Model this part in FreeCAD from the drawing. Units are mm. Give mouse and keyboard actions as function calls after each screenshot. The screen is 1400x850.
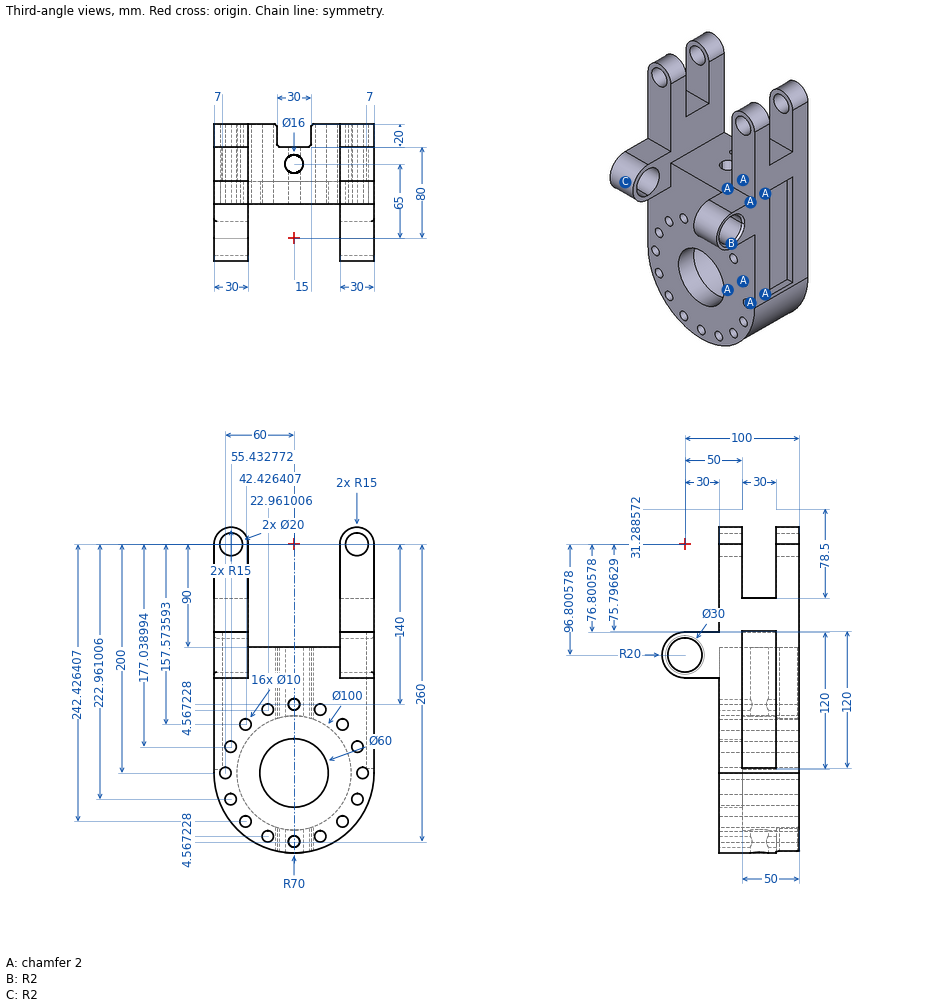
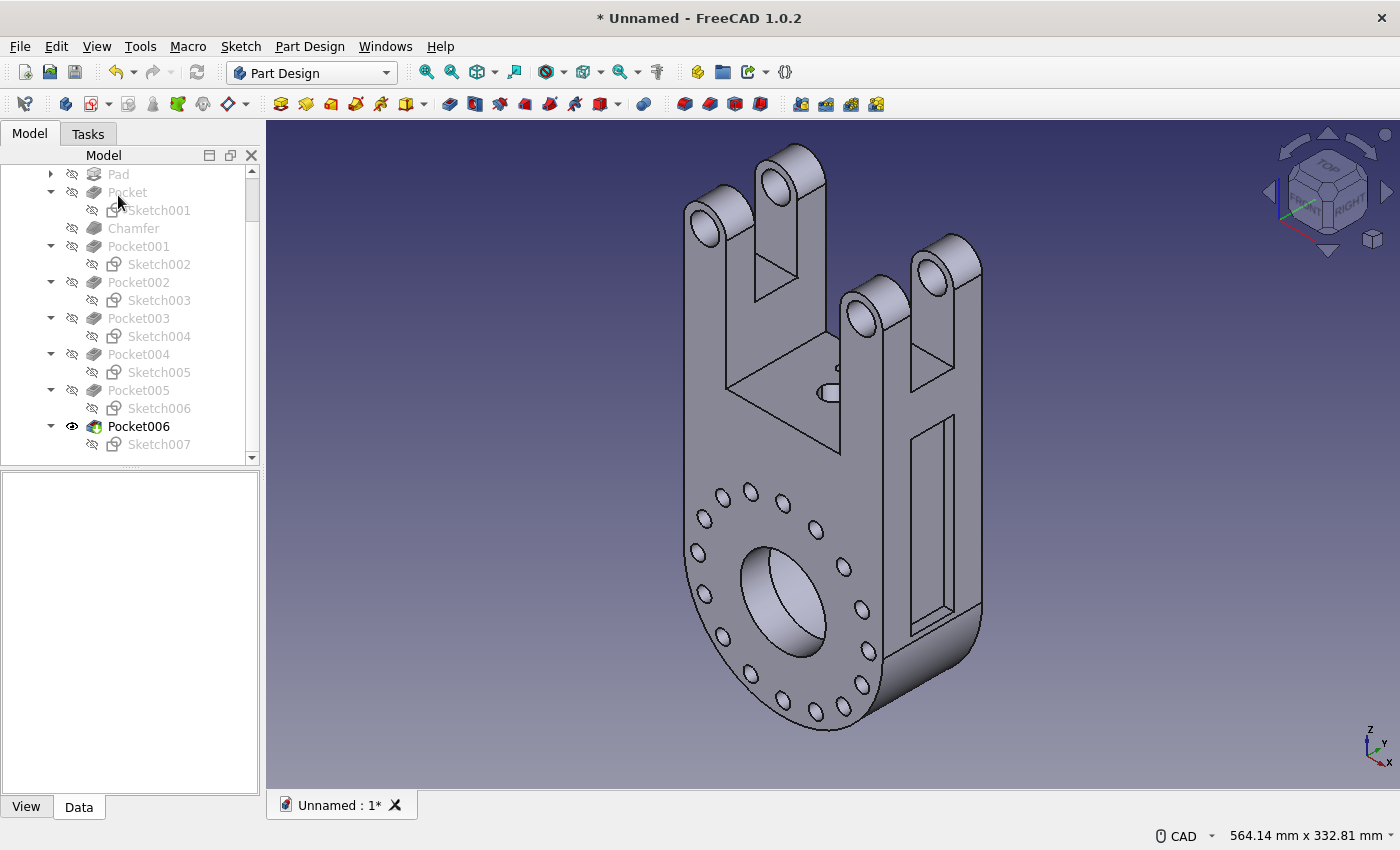
key(6)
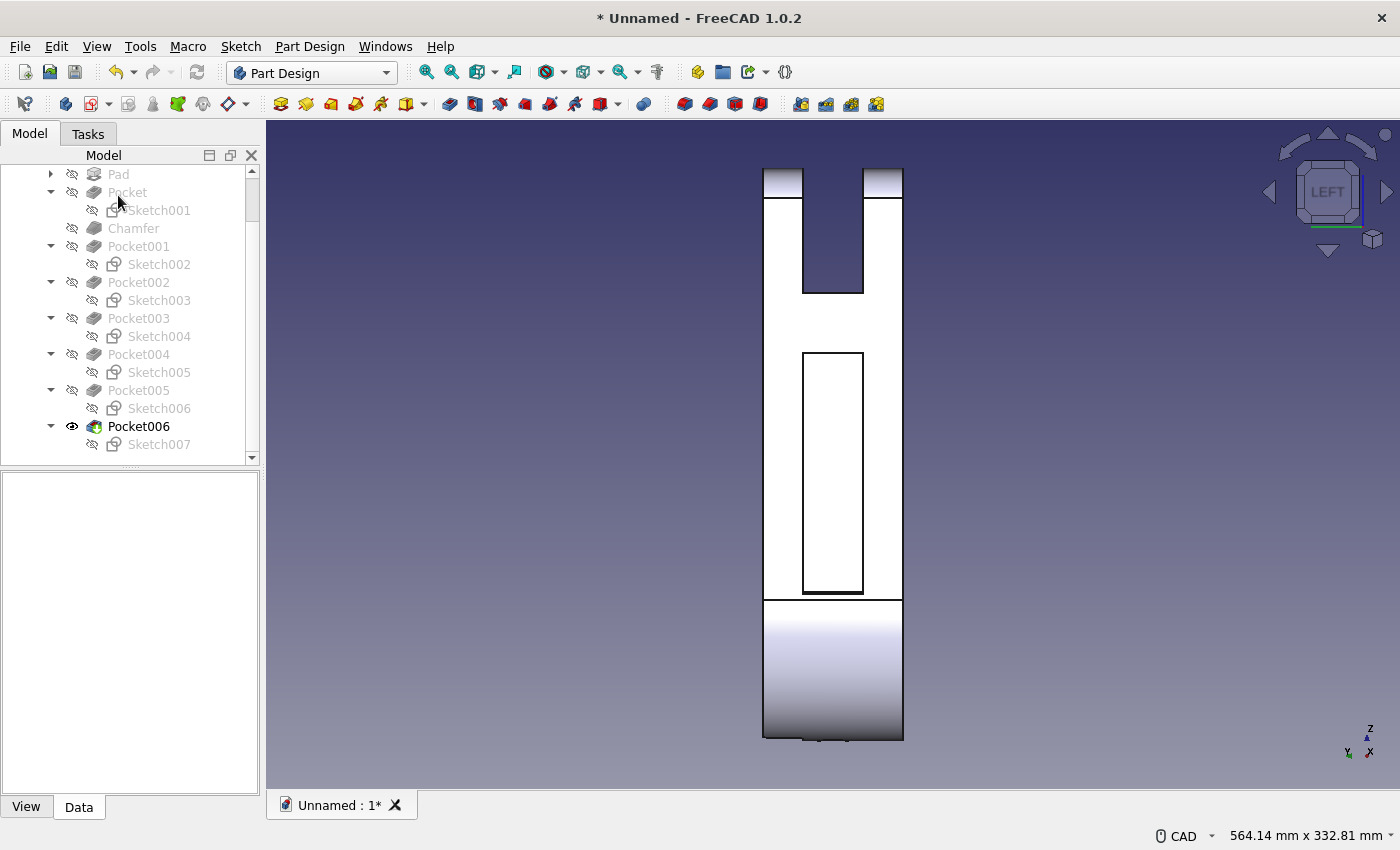
click(793, 341)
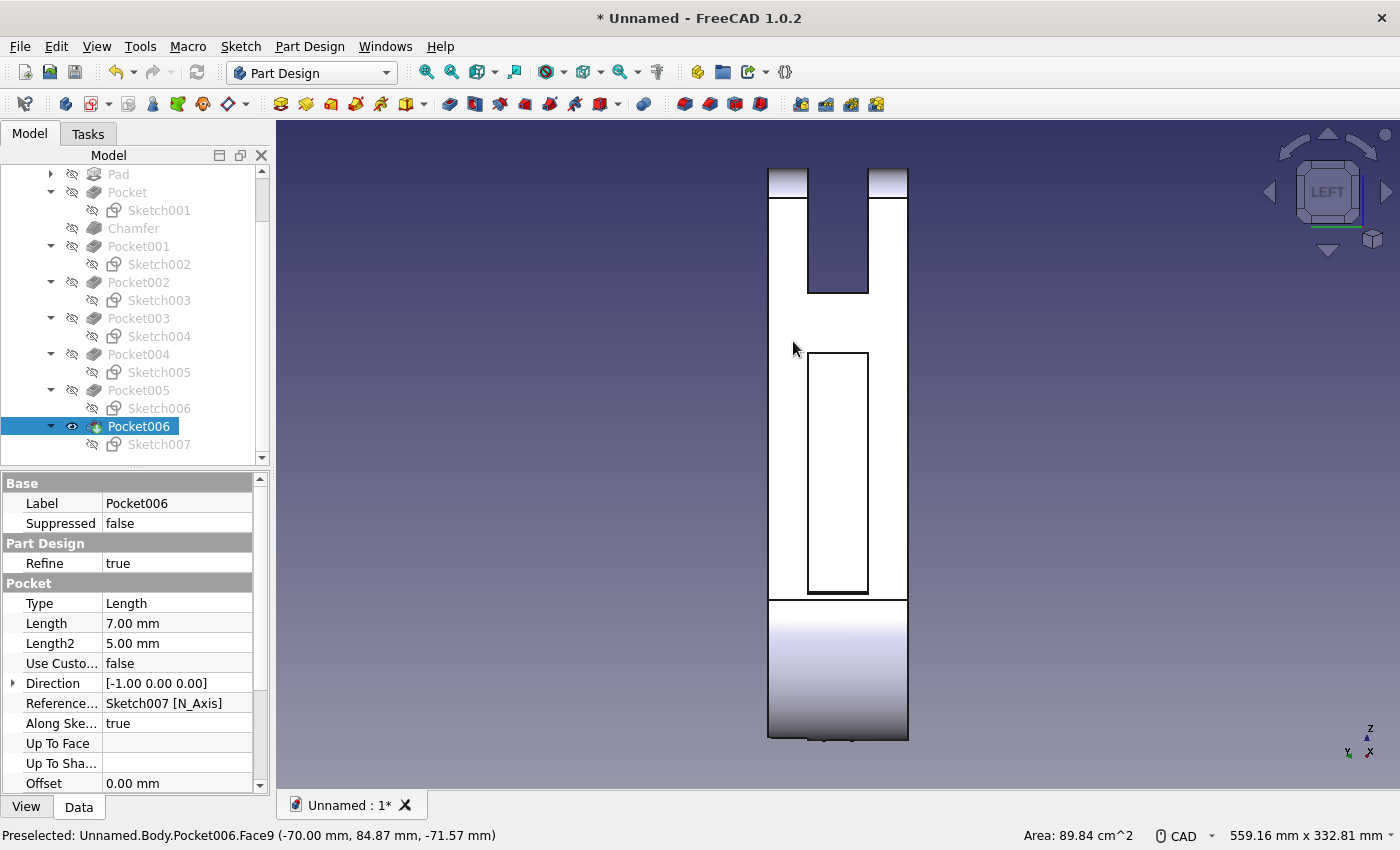
click(90, 104)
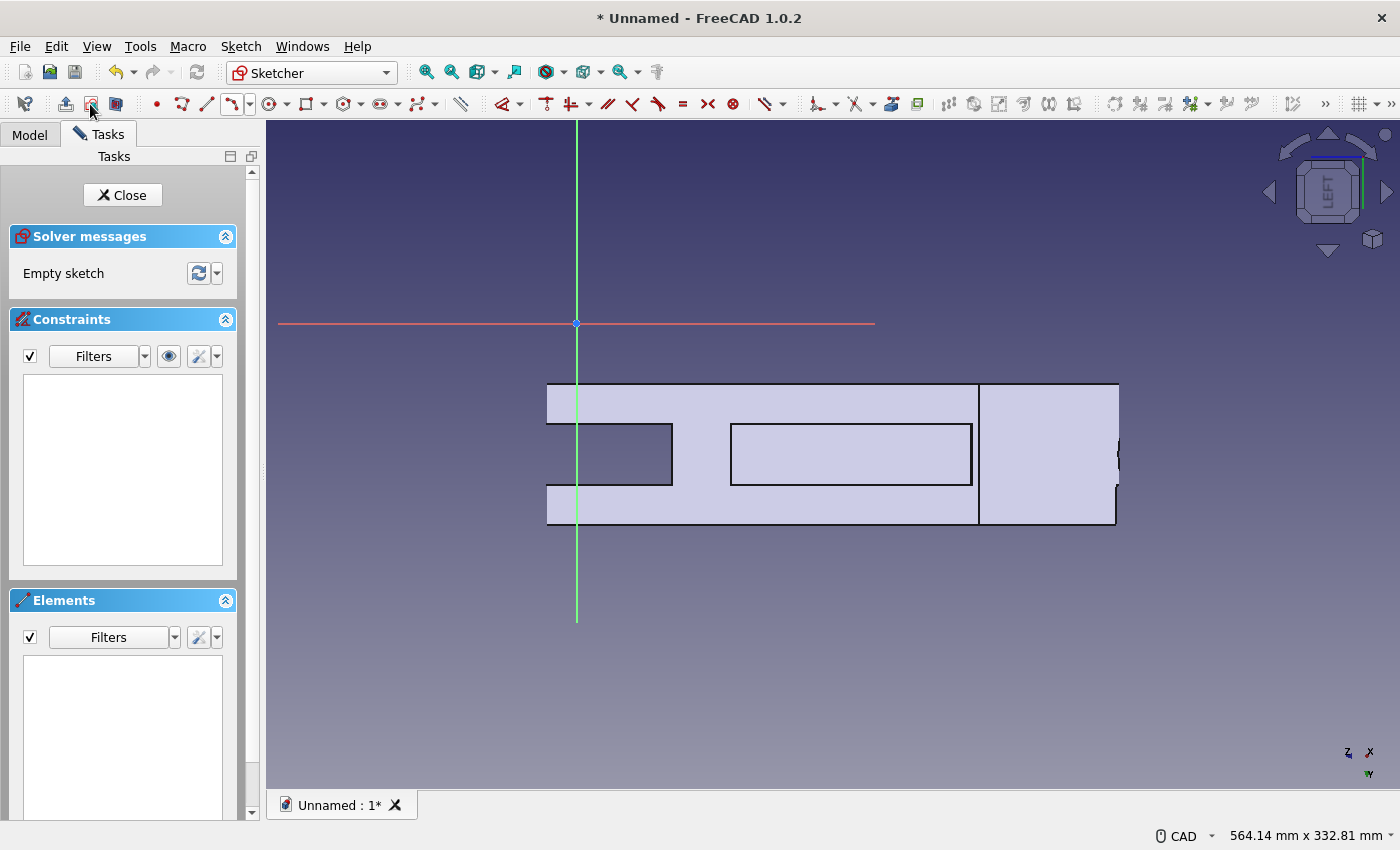
scroll(653, 296, up, 5)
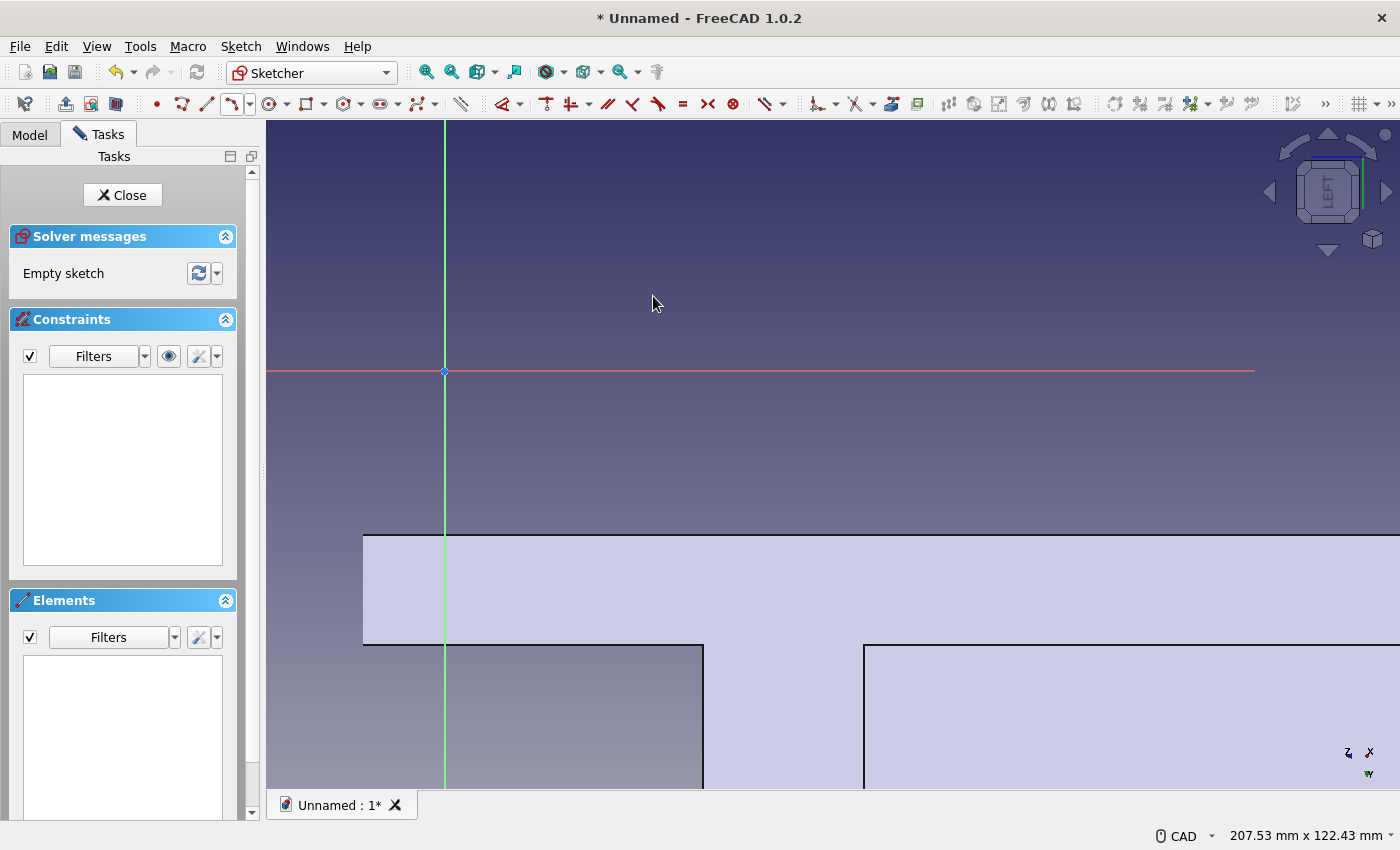
key(g)
key(m)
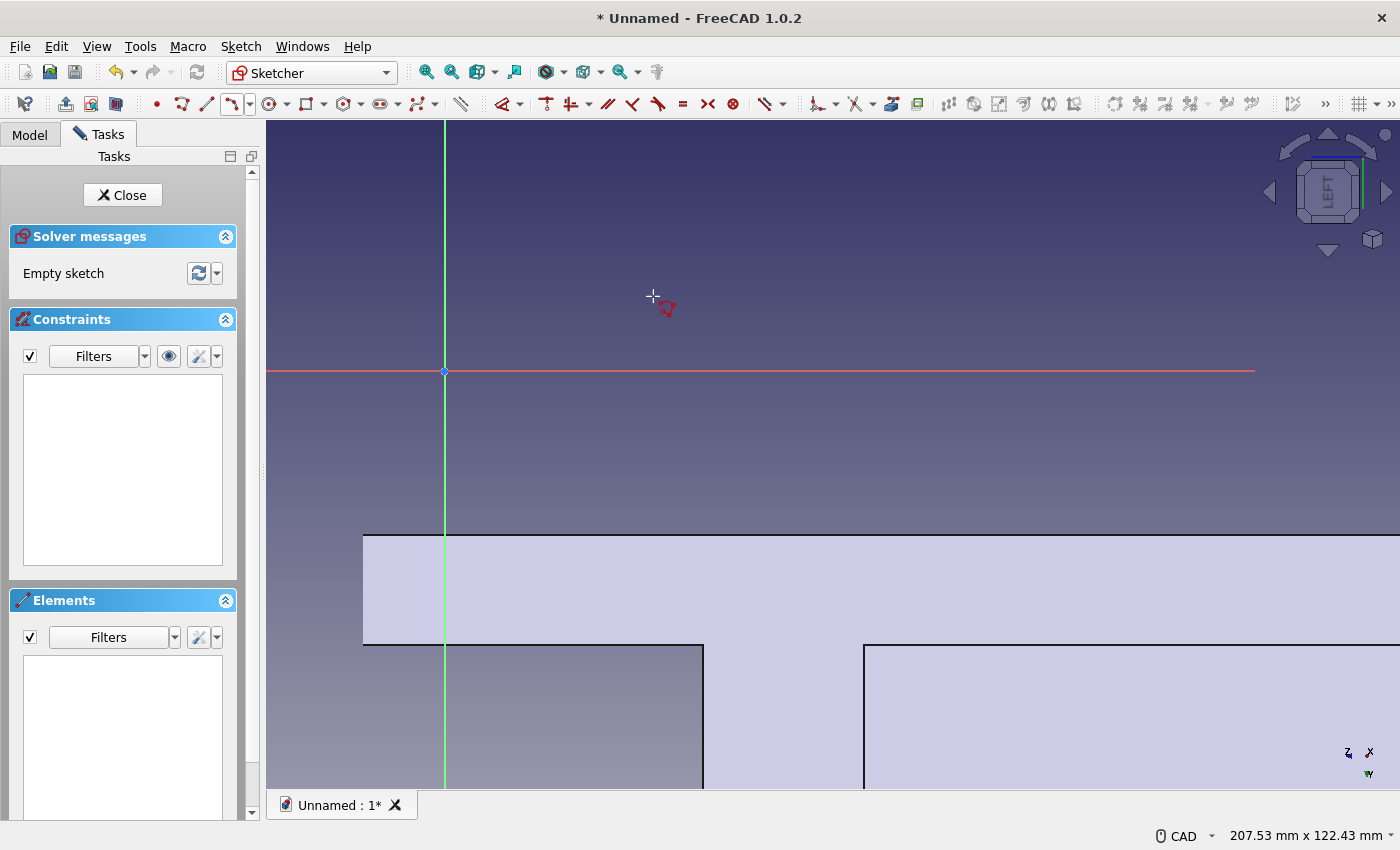
click(864, 371)
click(864, 645)
click(1083, 645)
click(1083, 371)
right_click(1083, 371)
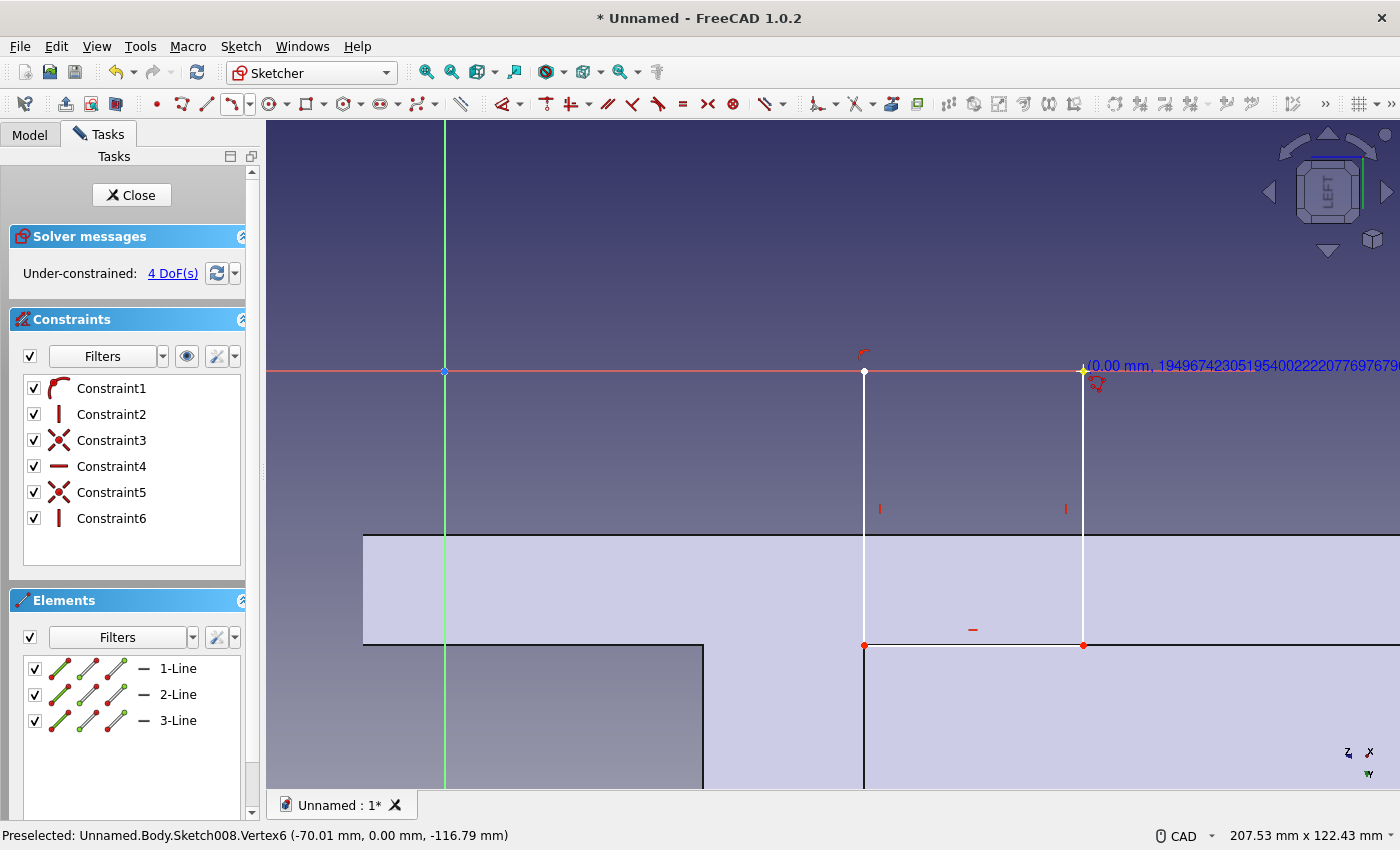
key(g)
key(3)
key(a)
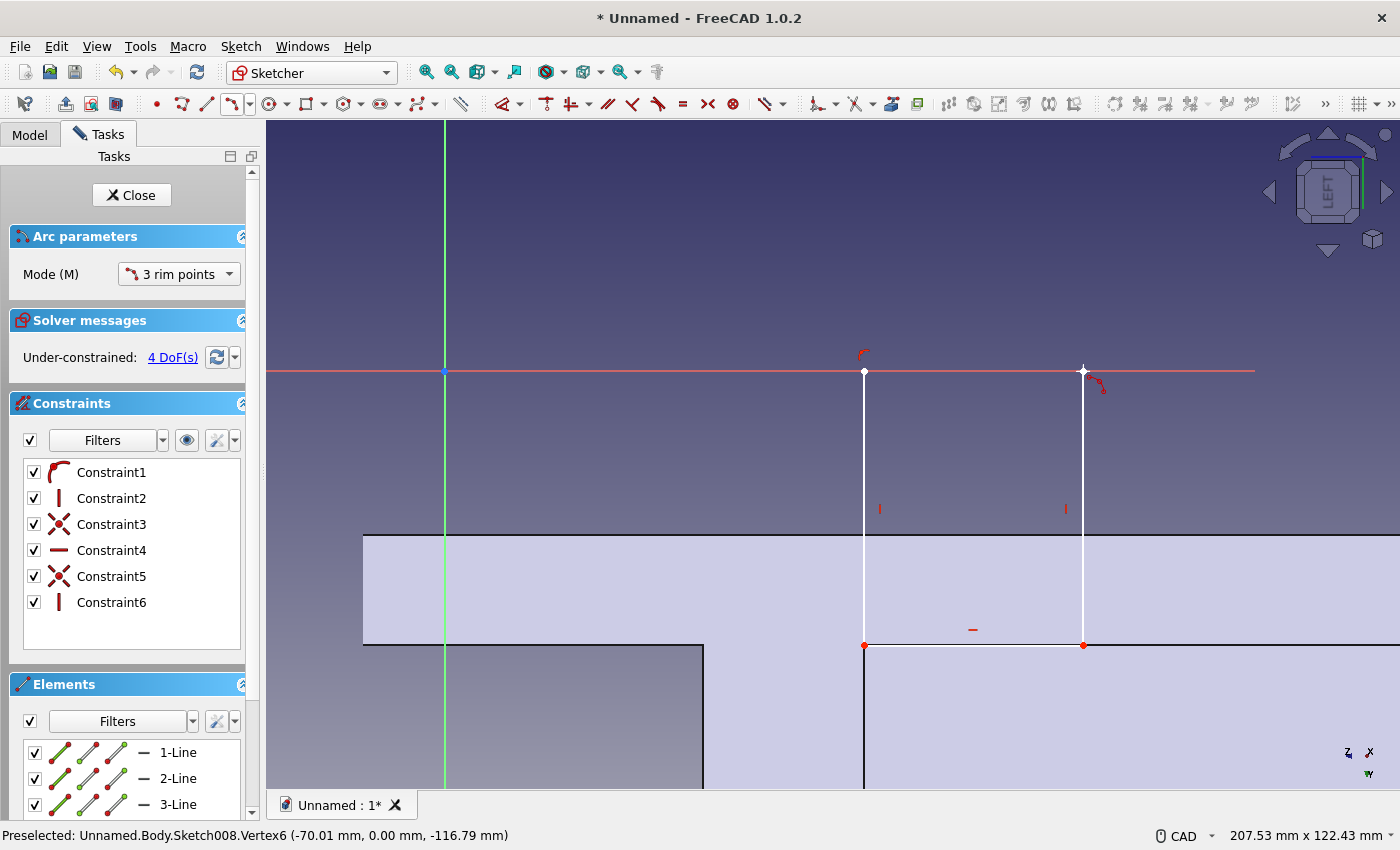
click(1083, 371)
click(864, 371)
click(974, 262)